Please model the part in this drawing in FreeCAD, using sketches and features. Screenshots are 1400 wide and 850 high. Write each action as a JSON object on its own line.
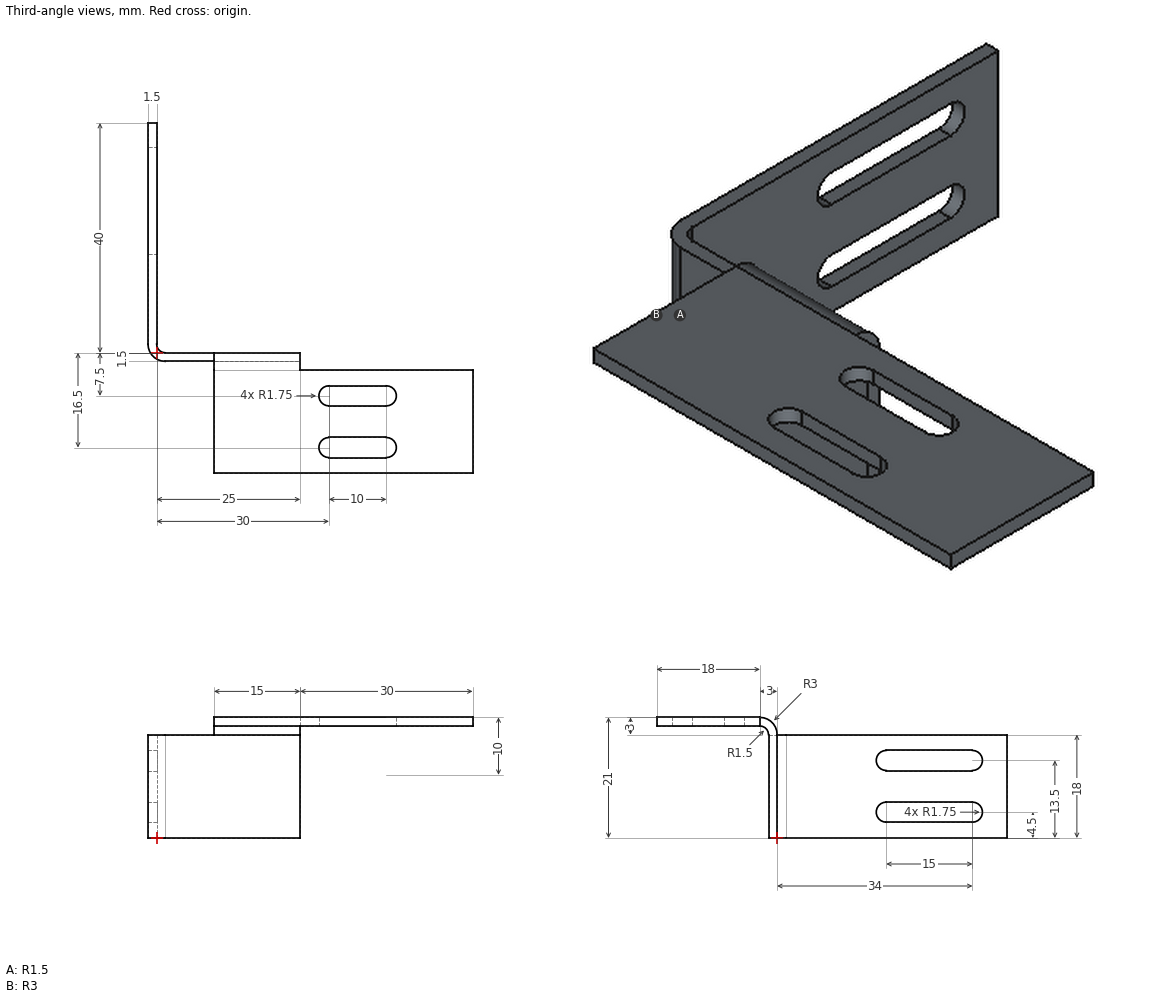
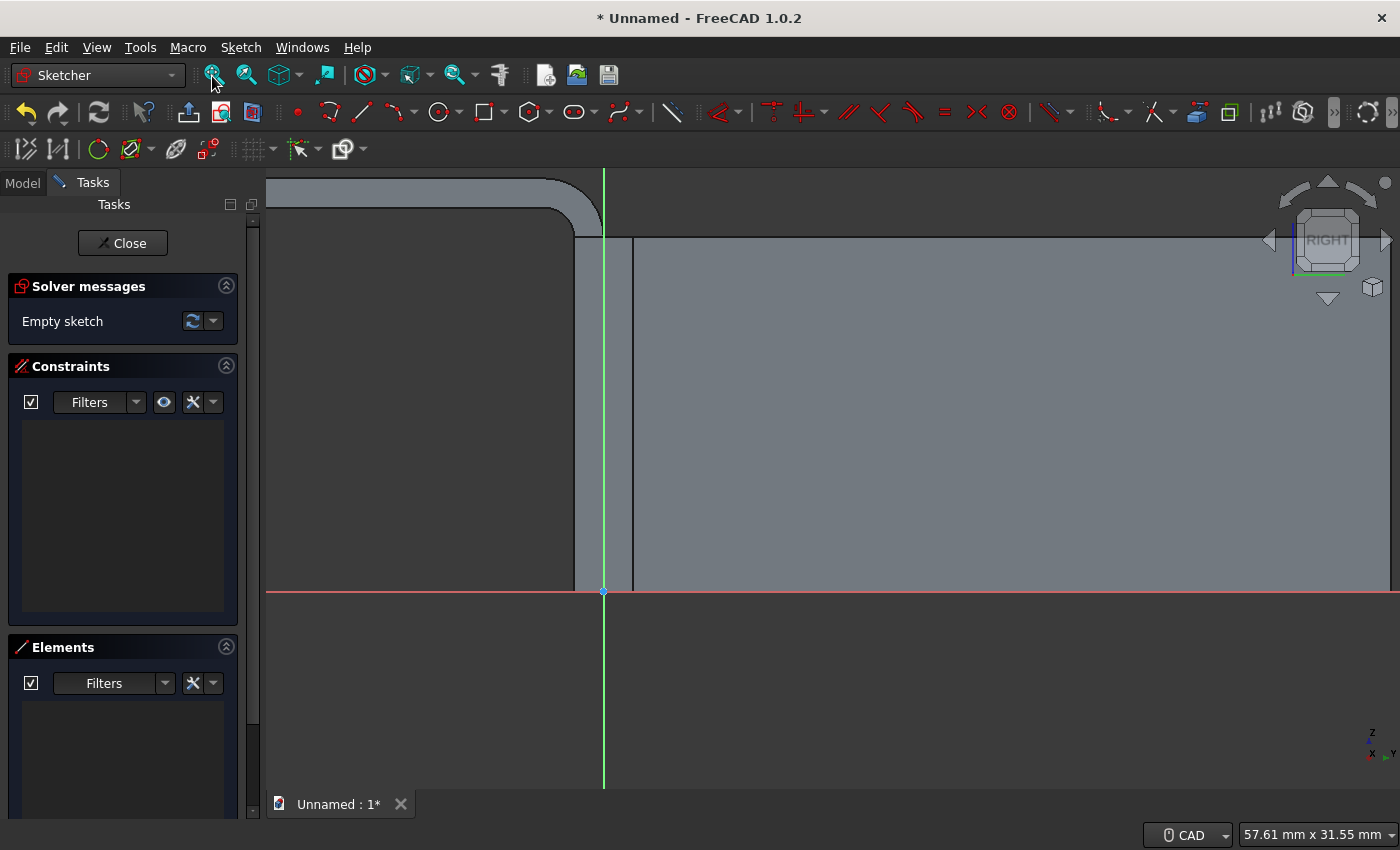
{"action": "scroll", "coordinate": [764, 478], "scroll_direction": "down", "scroll_amount": 5}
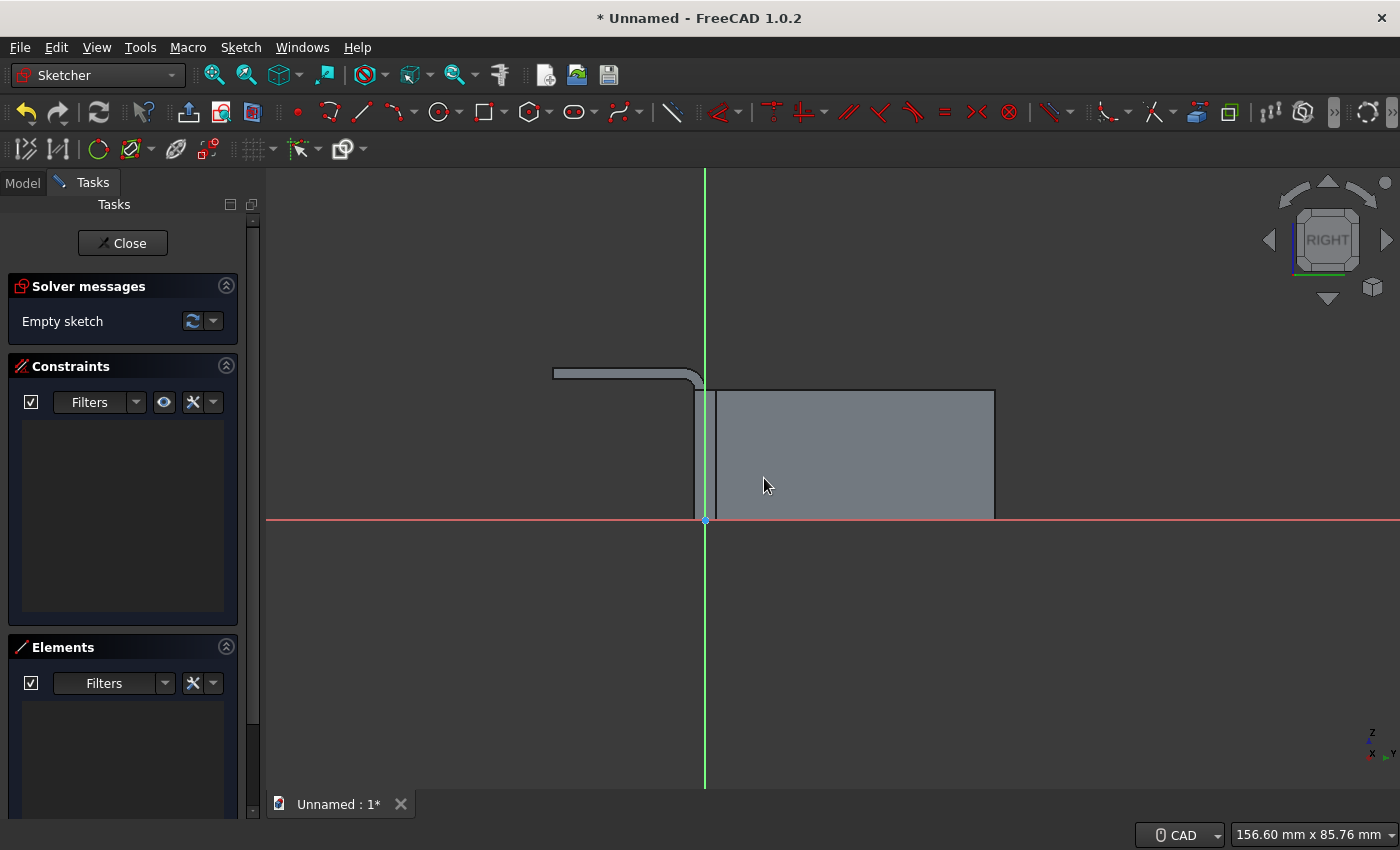
{"action": "scroll", "coordinate": [691, 374], "scroll_direction": "up", "scroll_amount": 15}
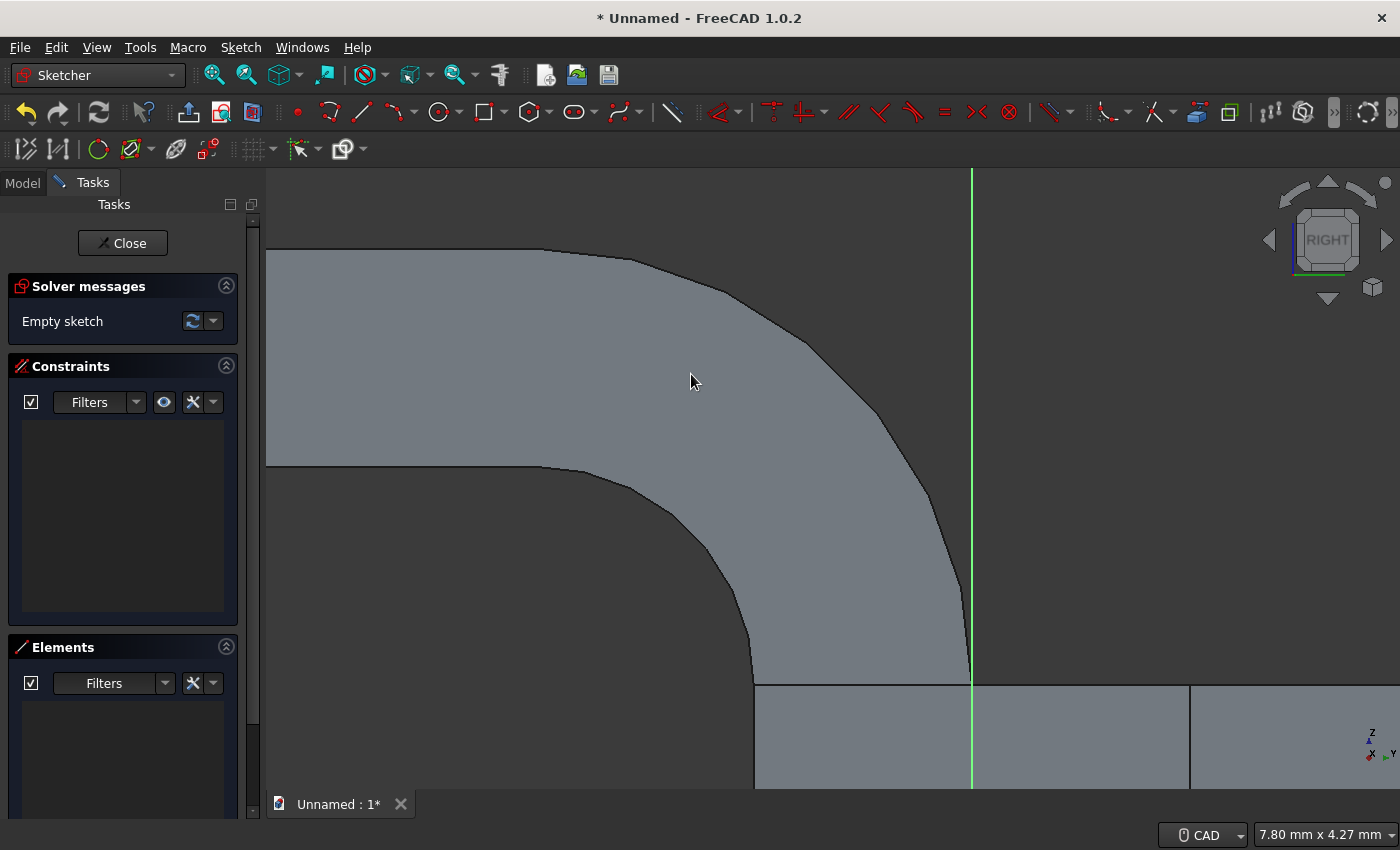
{"action": "left_click", "coordinate": [484, 112]}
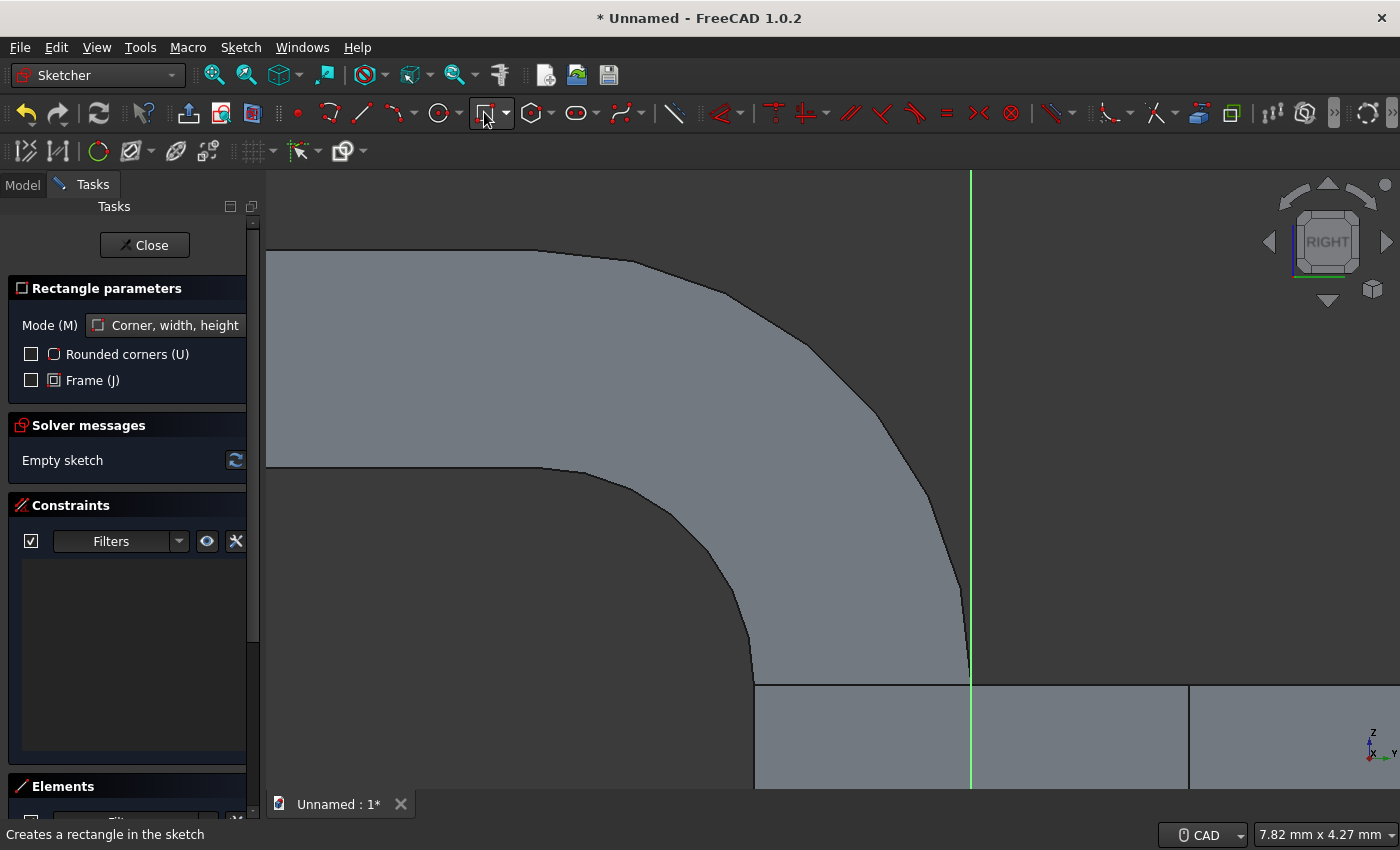
{"action": "left_click", "coordinate": [537, 250]}
{"action": "left_click", "coordinate": [971, 685]}
{"action": "key", "text": "Escape"}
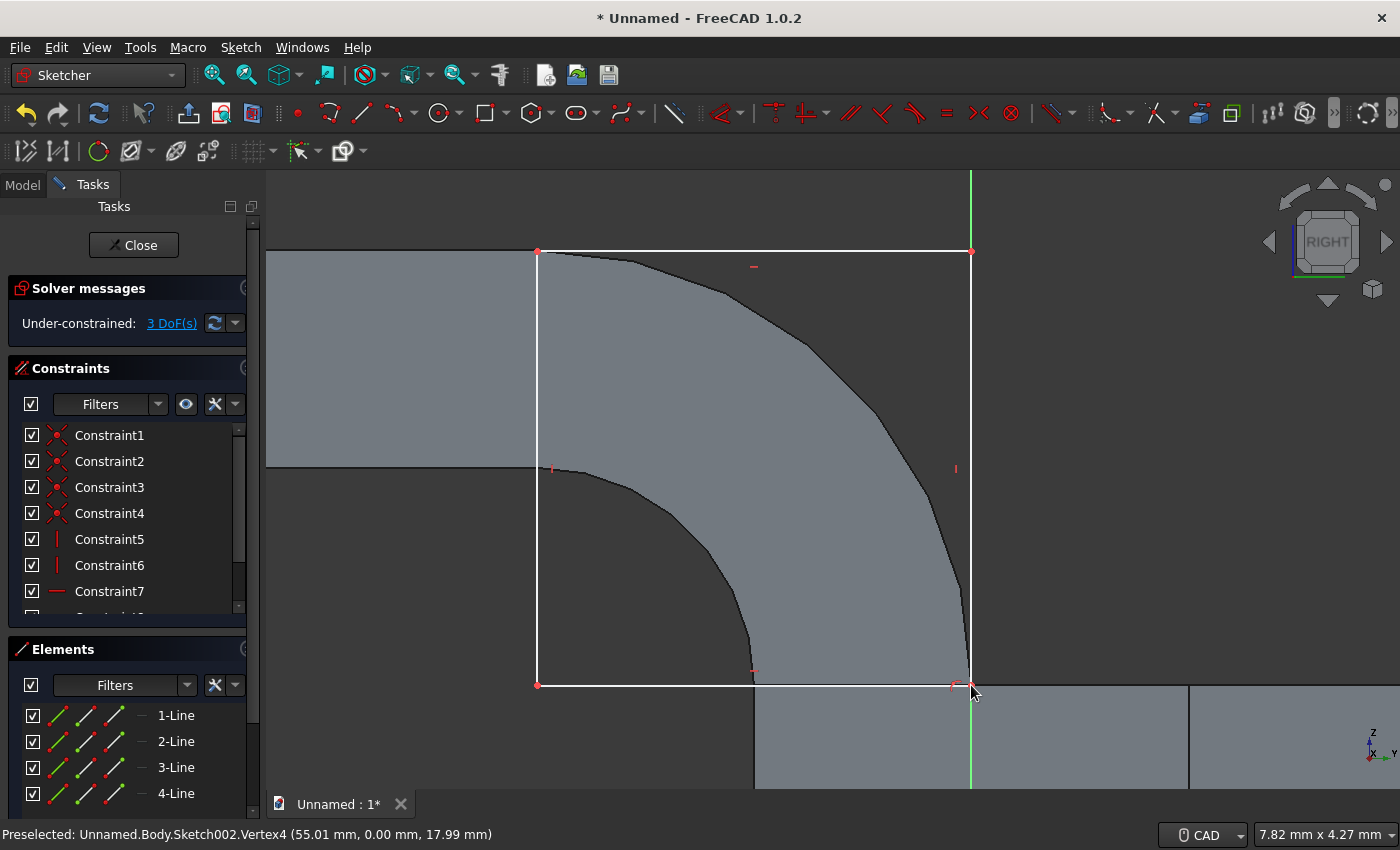
{"action": "key", "text": "d"}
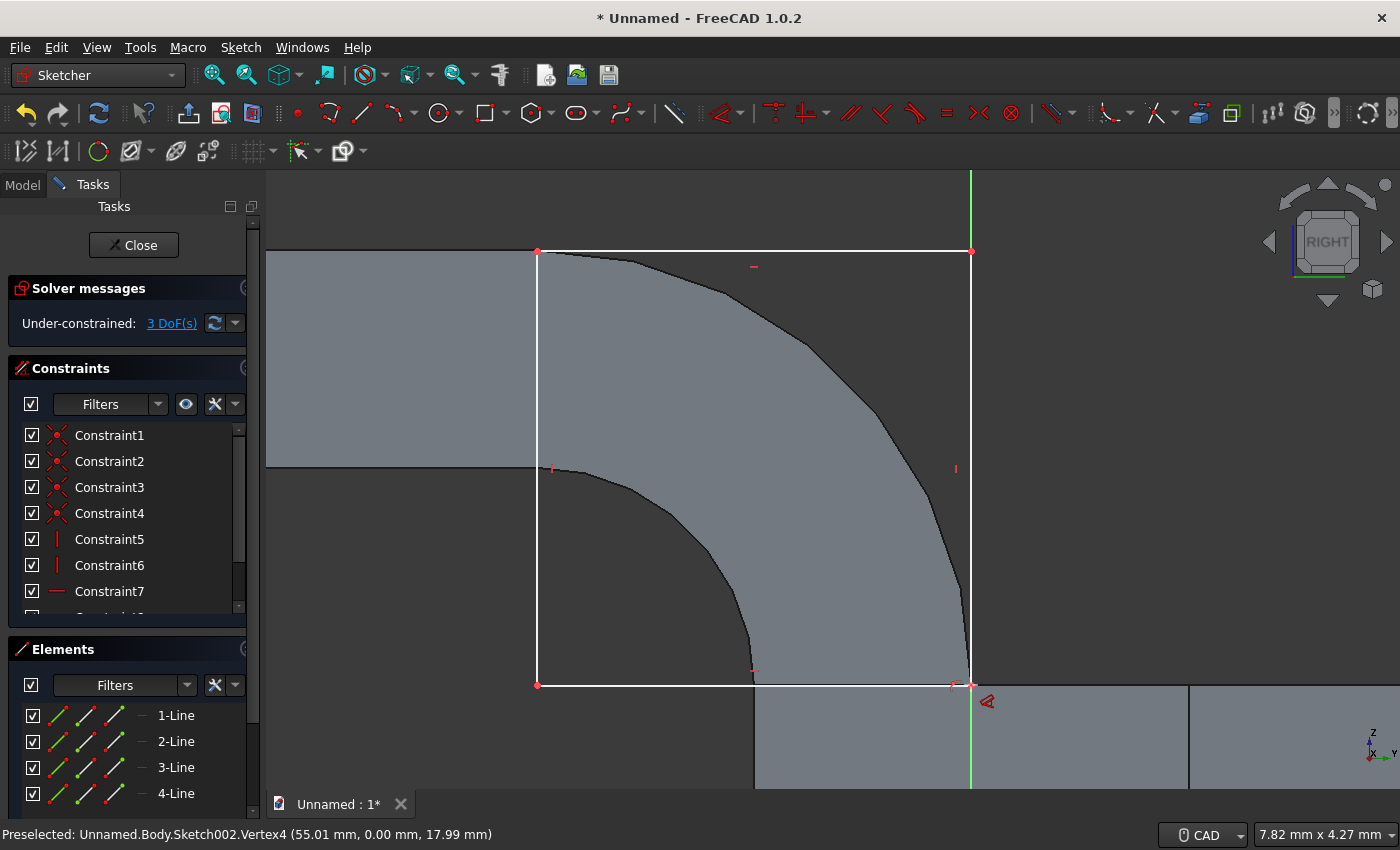
{"action": "left_click", "coordinate": [537, 381]}
{"action": "left_click", "coordinate": [503, 468]}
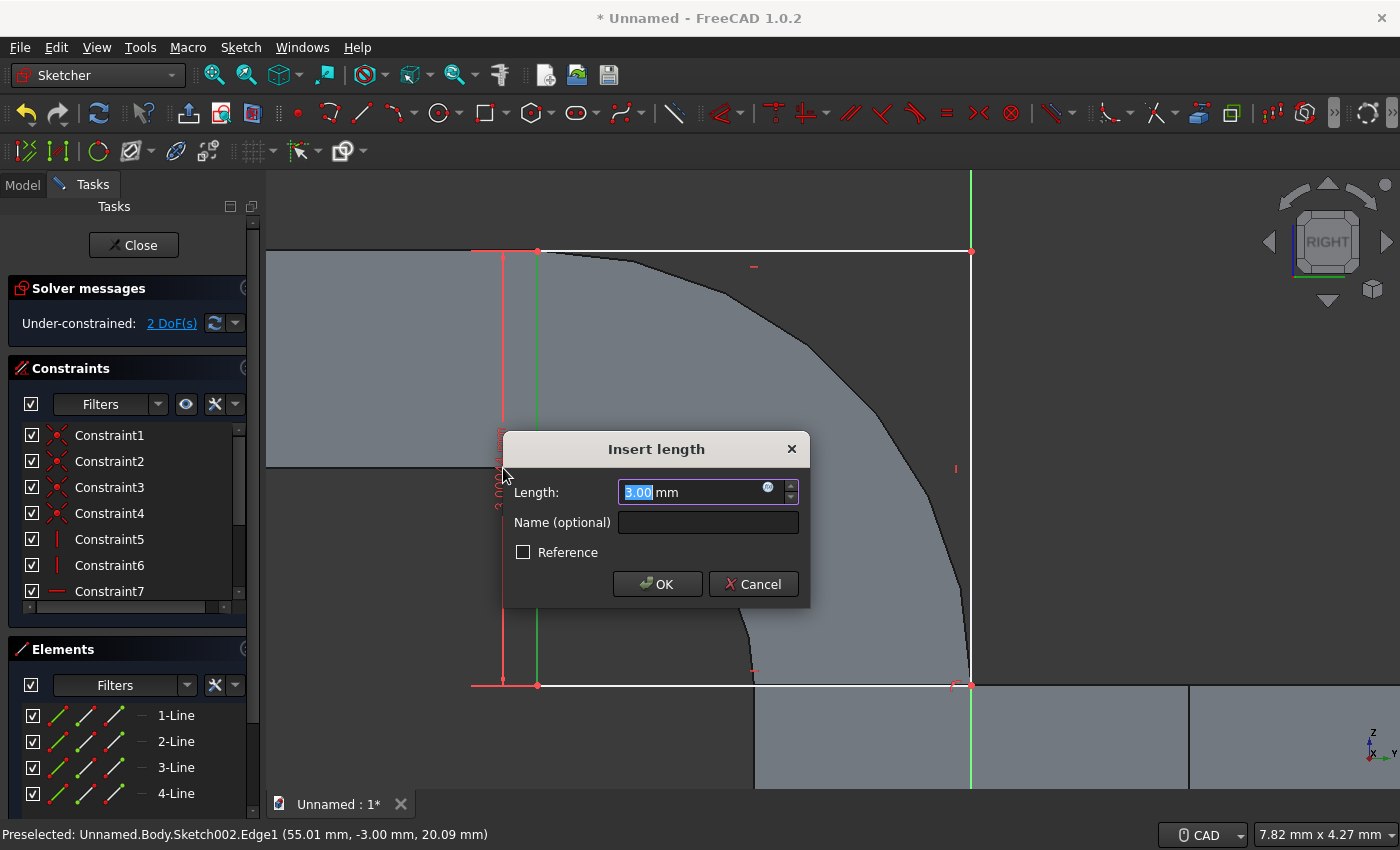
{"action": "type", "text": "3"}
{"action": "key", "text": "Return"}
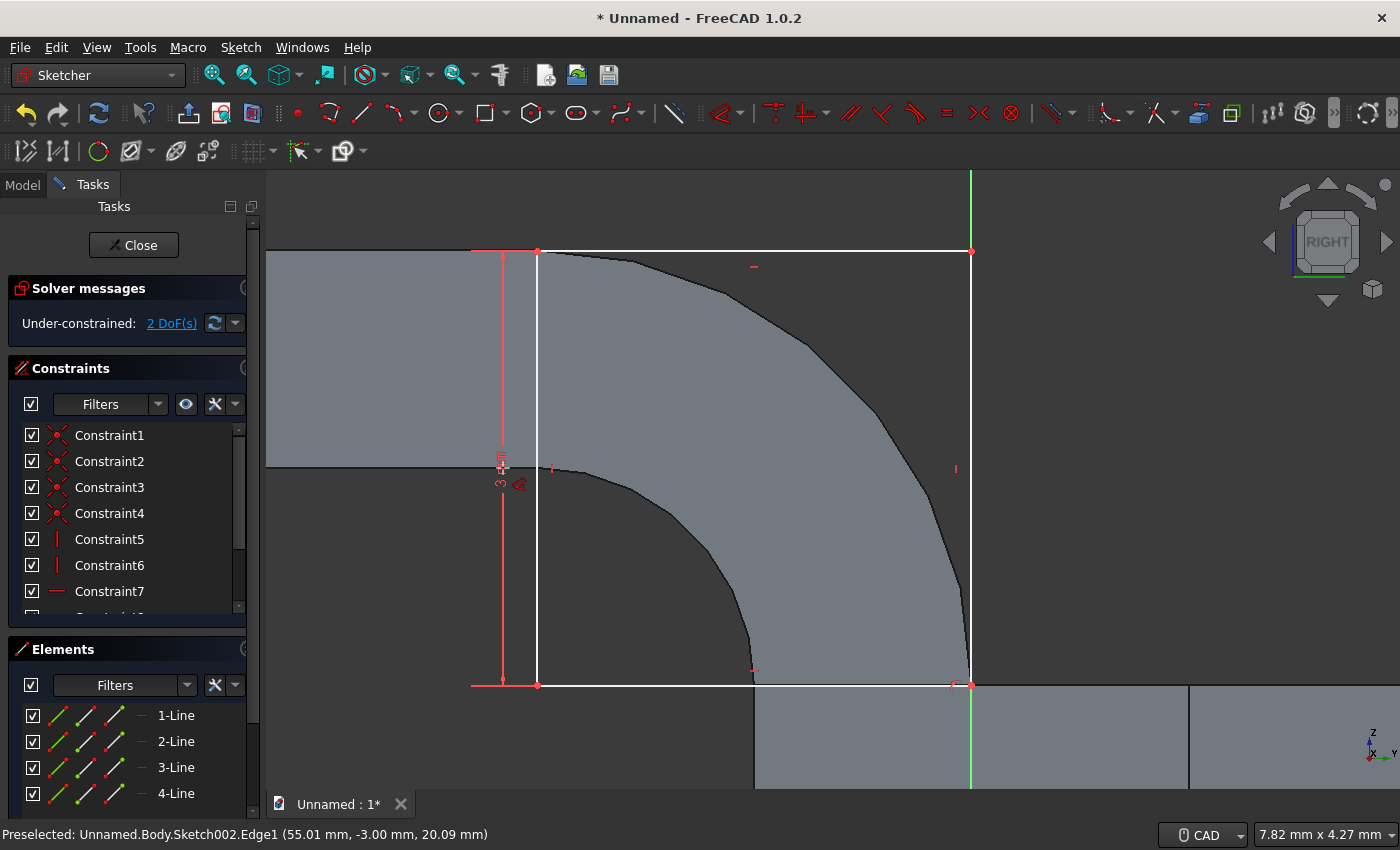
{"action": "left_click", "coordinate": [667, 686]}
{"action": "left_click", "coordinate": [754, 720]}